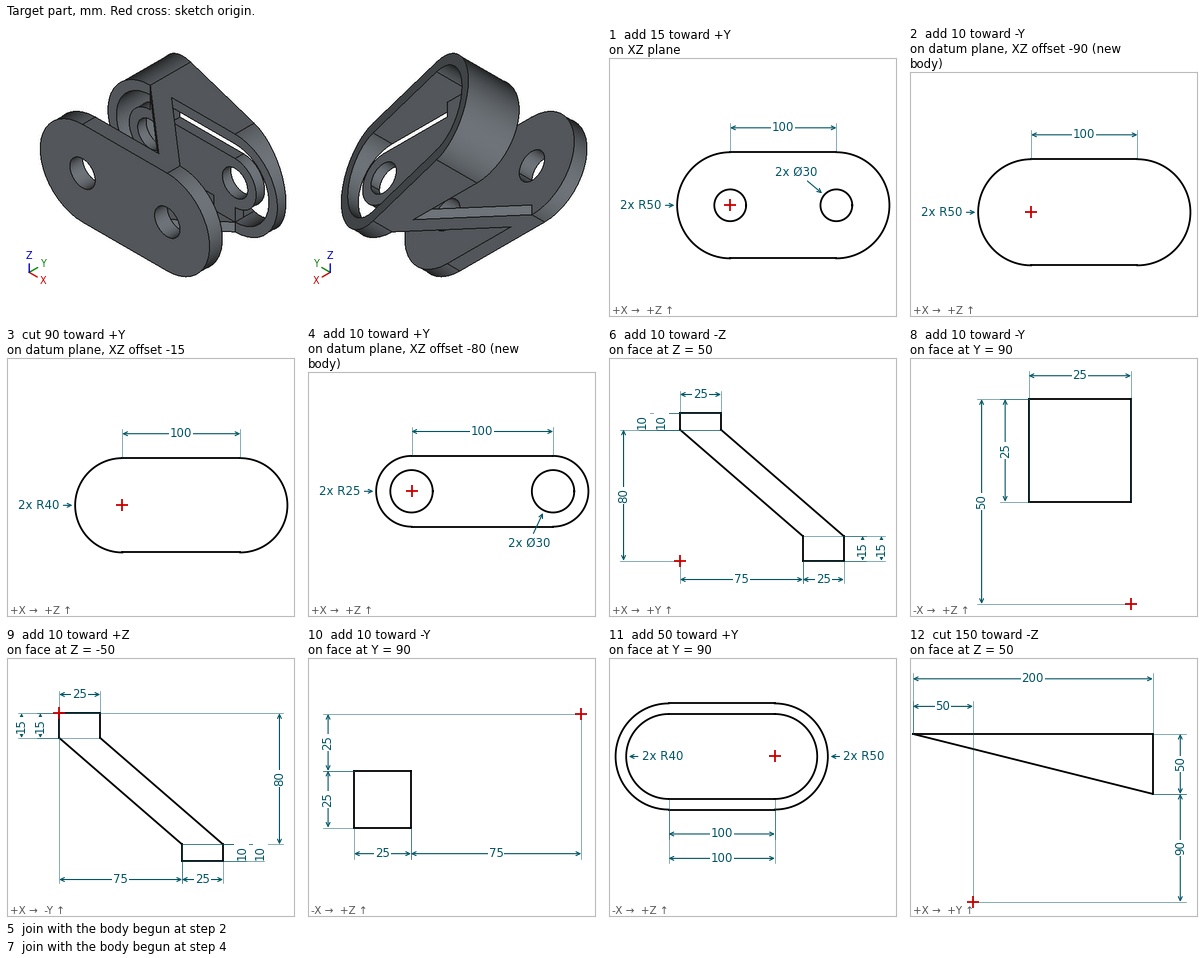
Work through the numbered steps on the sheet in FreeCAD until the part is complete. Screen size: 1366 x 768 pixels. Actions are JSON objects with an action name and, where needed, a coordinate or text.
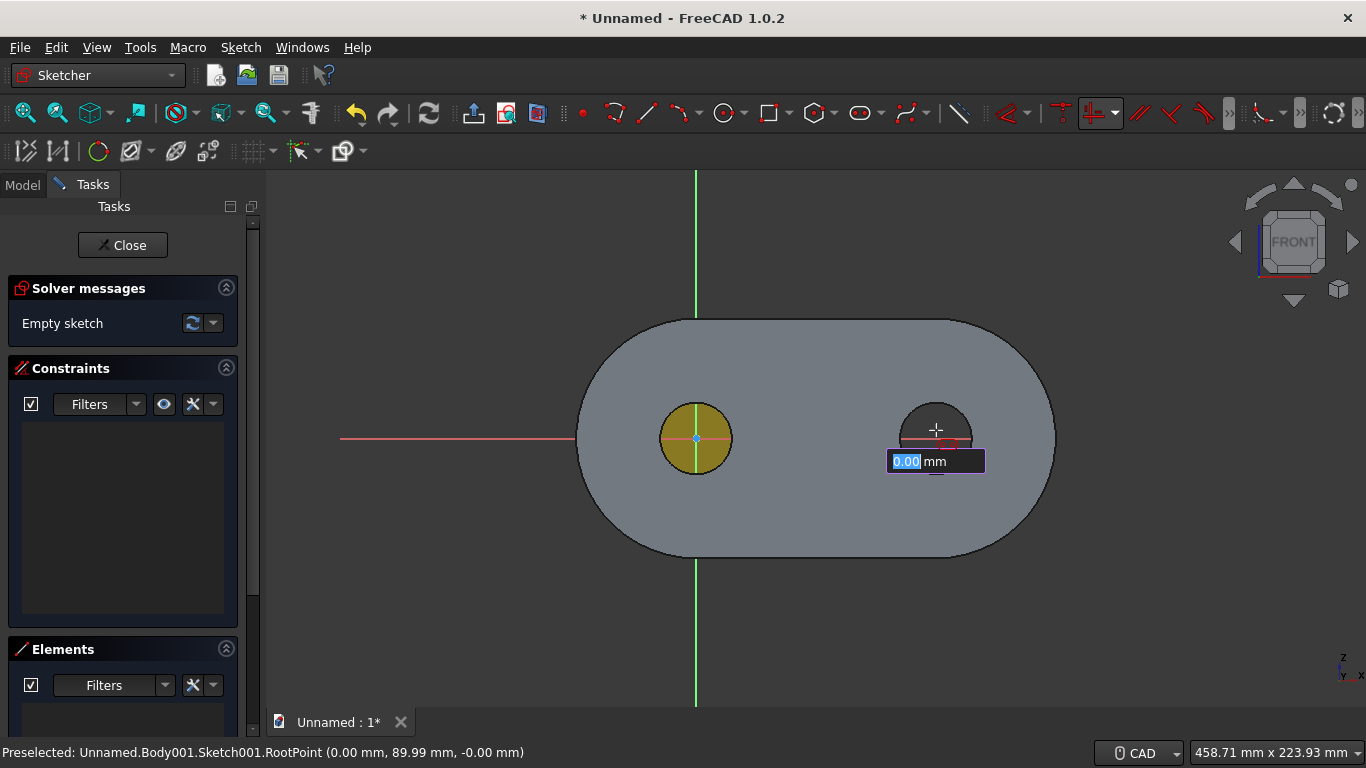
{"action": "left_click", "coordinate": [816, 558]}
{"action": "key", "text": "Escape"}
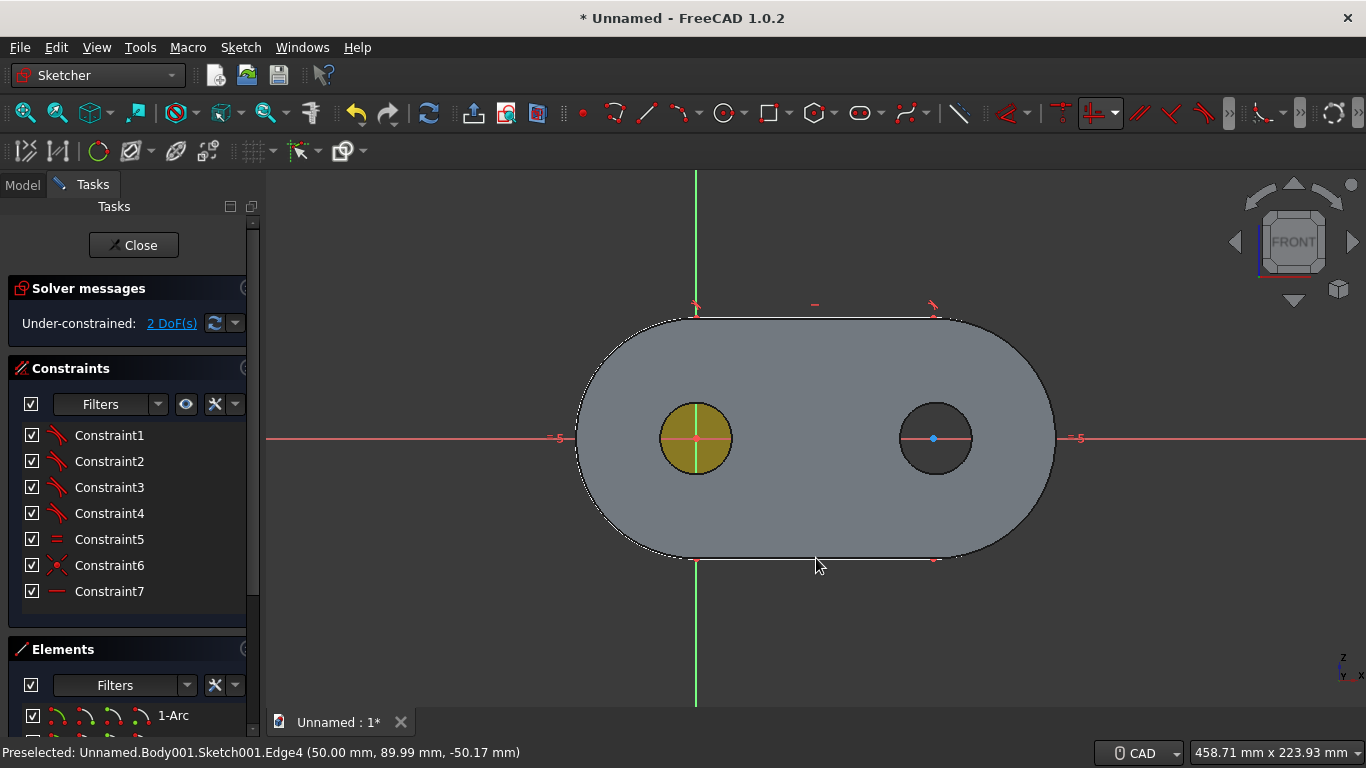
{"action": "left_click", "coordinate": [1006, 114]}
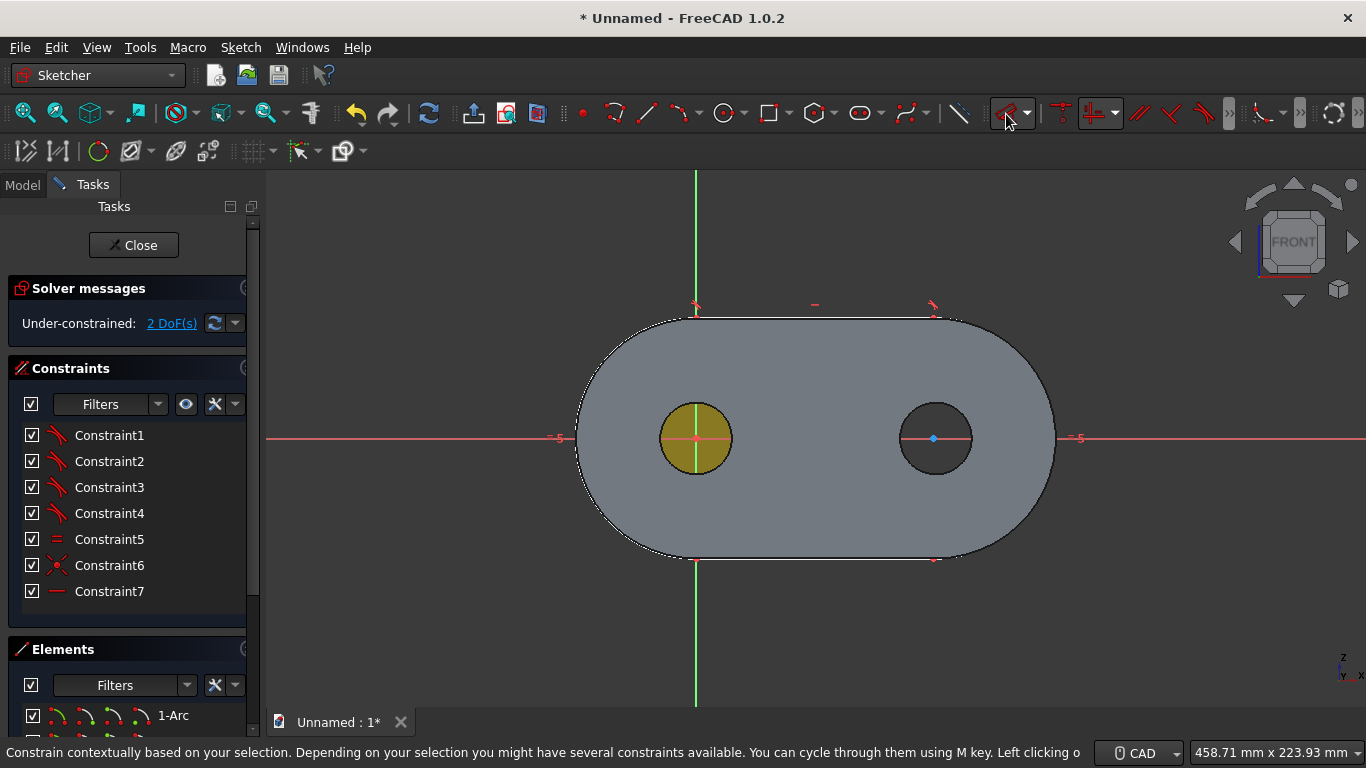
{"action": "left_click", "coordinate": [599, 368]}
{"action": "left_click", "coordinate": [573, 349]}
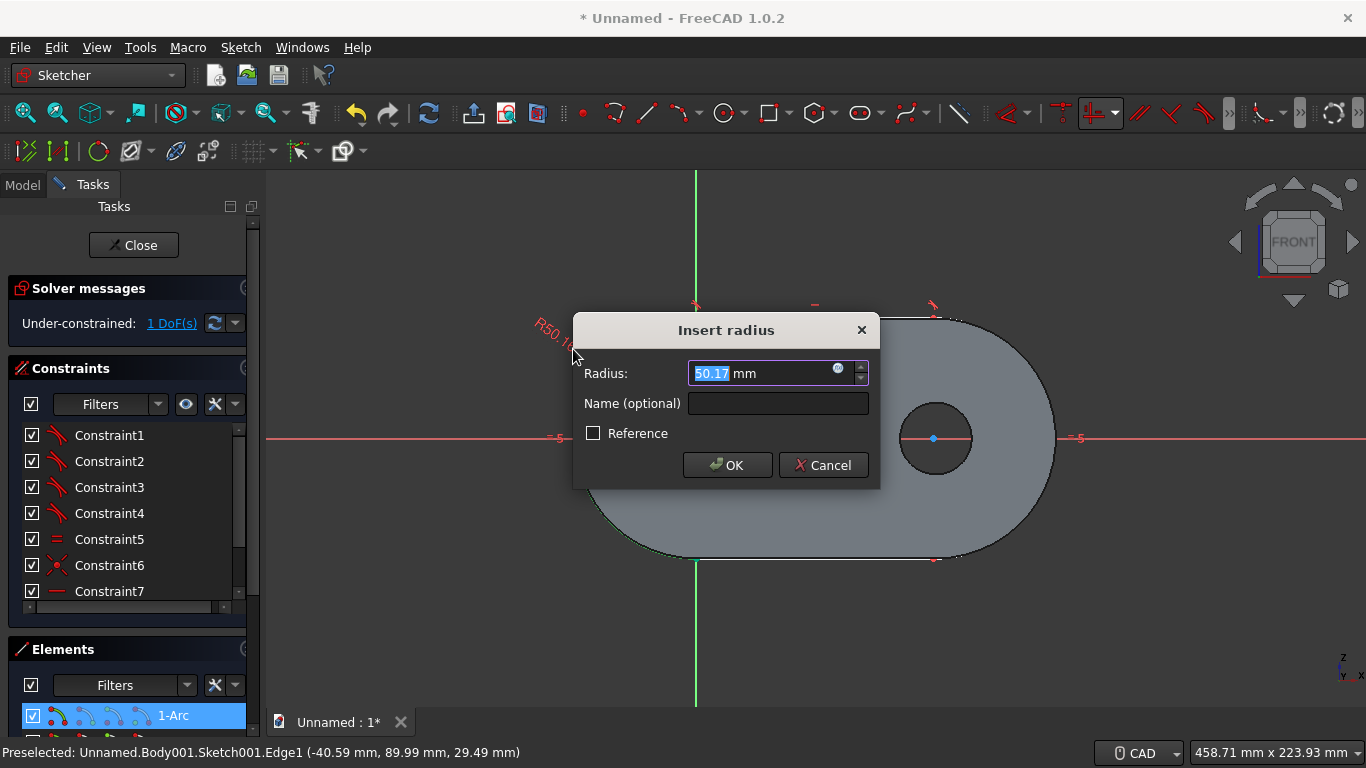
{"action": "type", "text": "50"}
{"action": "key", "text": "Return"}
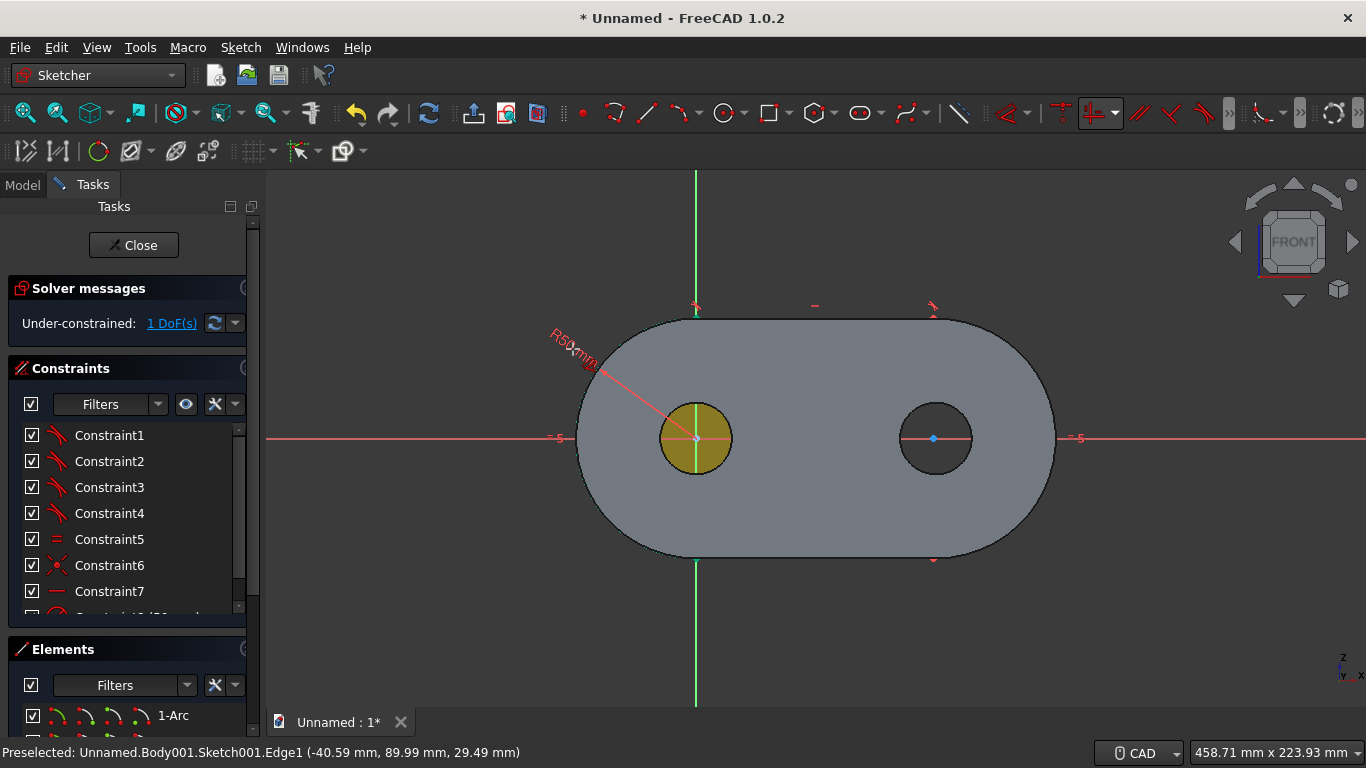
{"action": "left_click", "coordinate": [767, 319]}
{"action": "left_click", "coordinate": [815, 285]}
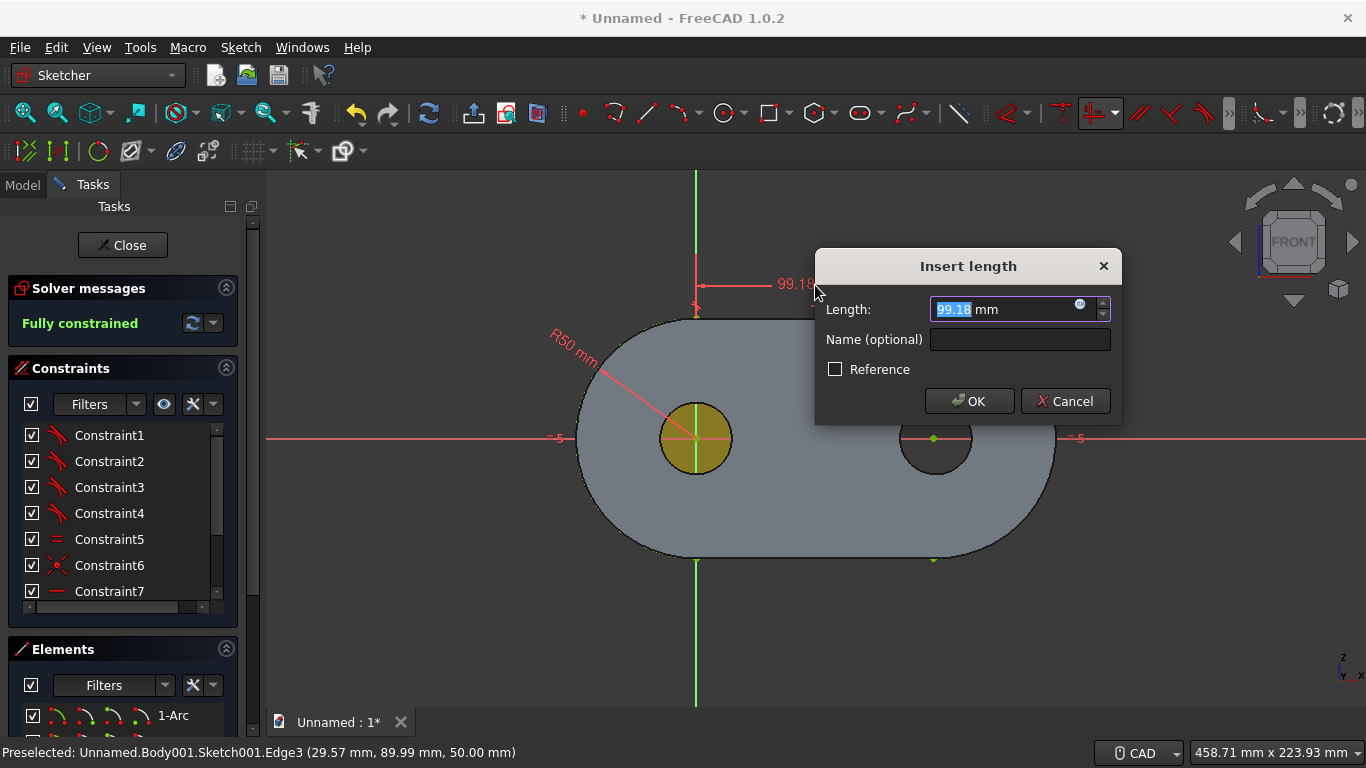
{"action": "type", "text": "100"}
{"action": "key", "text": "Return"}
{"action": "key", "text": "Escape"}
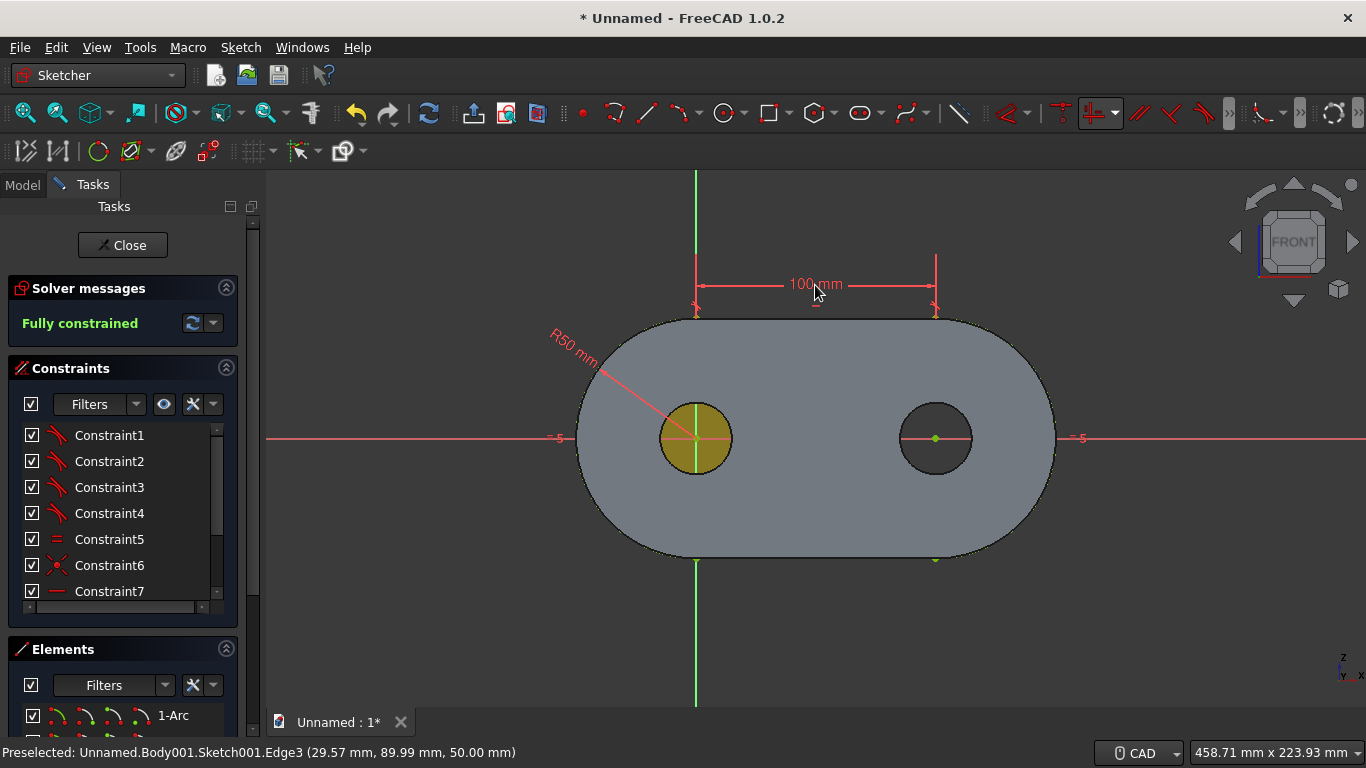
{"action": "left_click", "coordinate": [123, 245]}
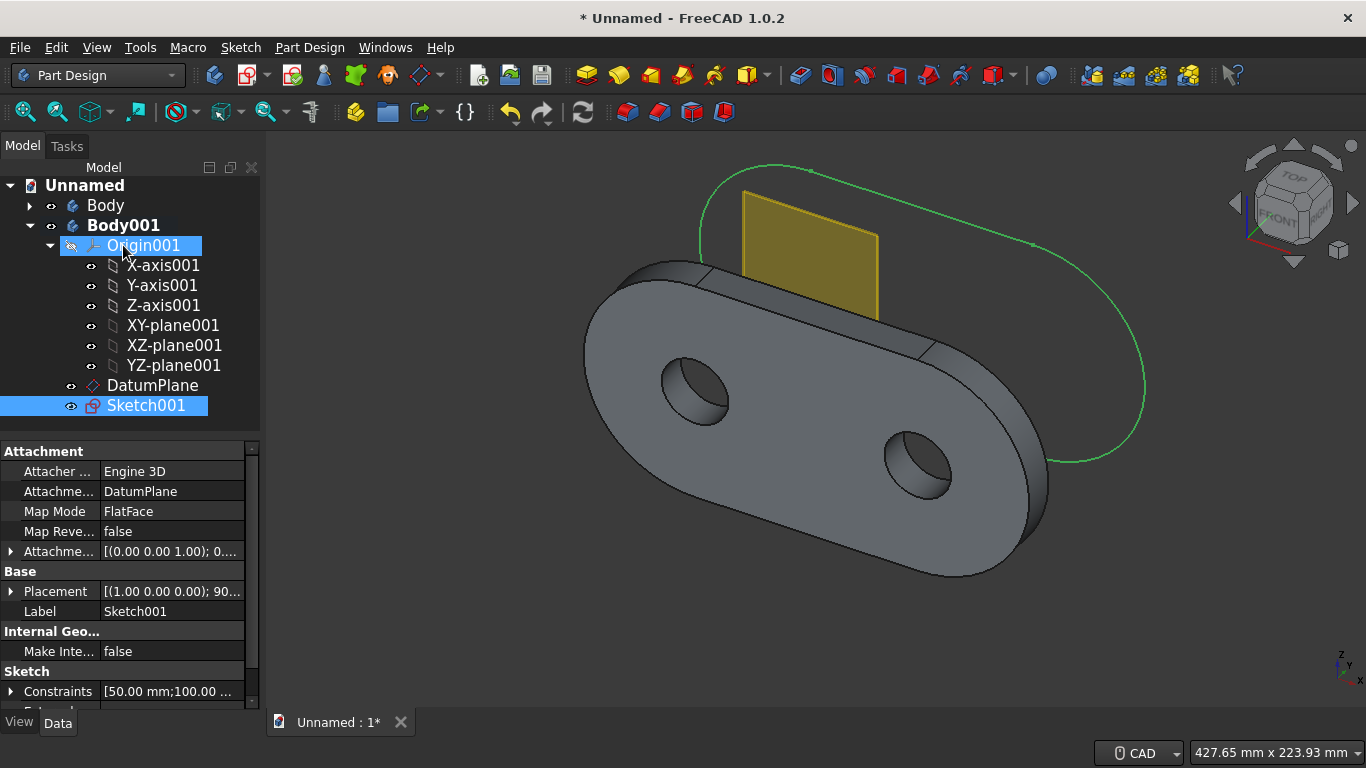
{"action": "left_click", "coordinate": [588, 76]}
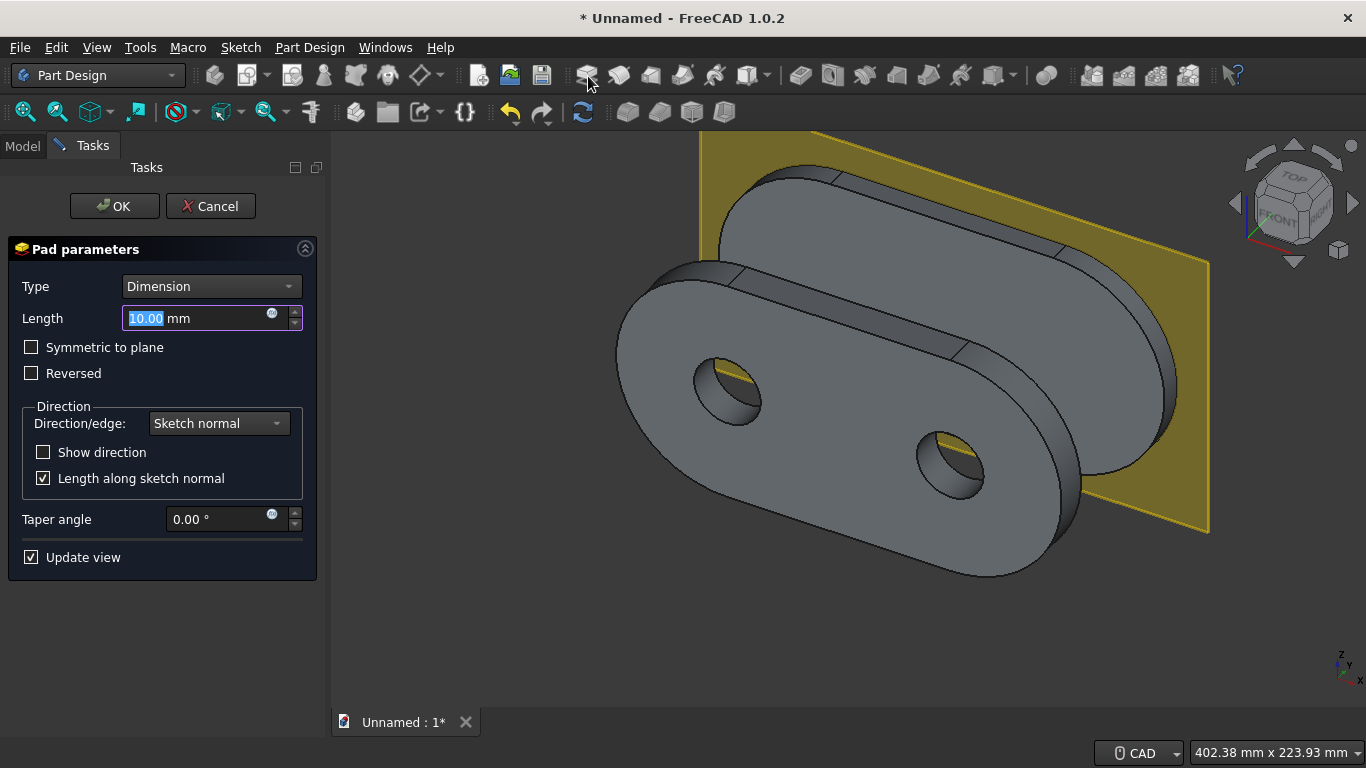
{"action": "type", "text": "10"}
{"action": "key", "text": "Tab"}